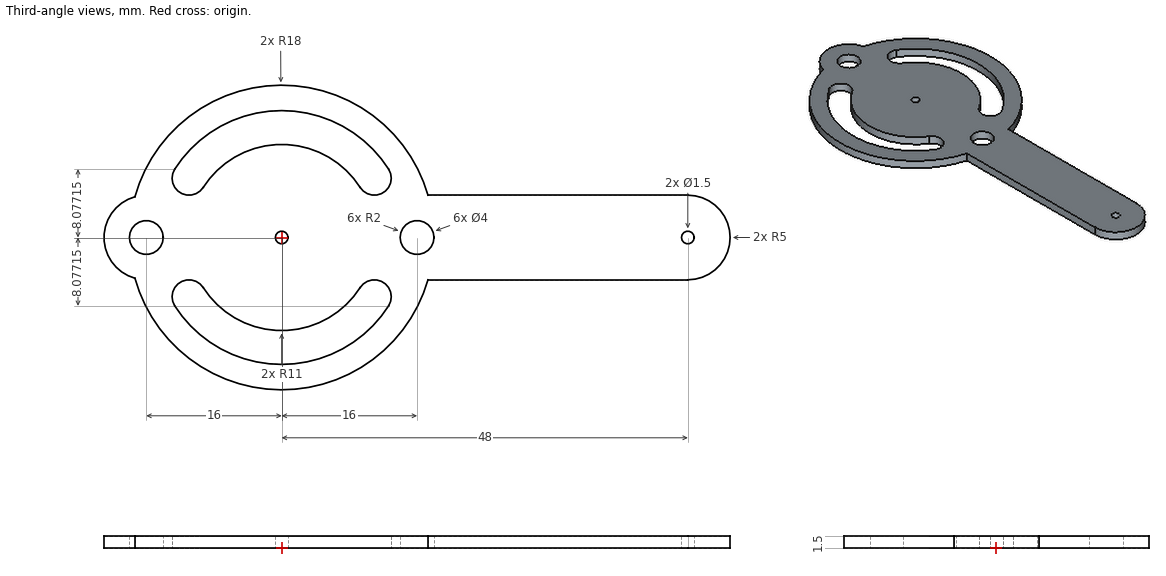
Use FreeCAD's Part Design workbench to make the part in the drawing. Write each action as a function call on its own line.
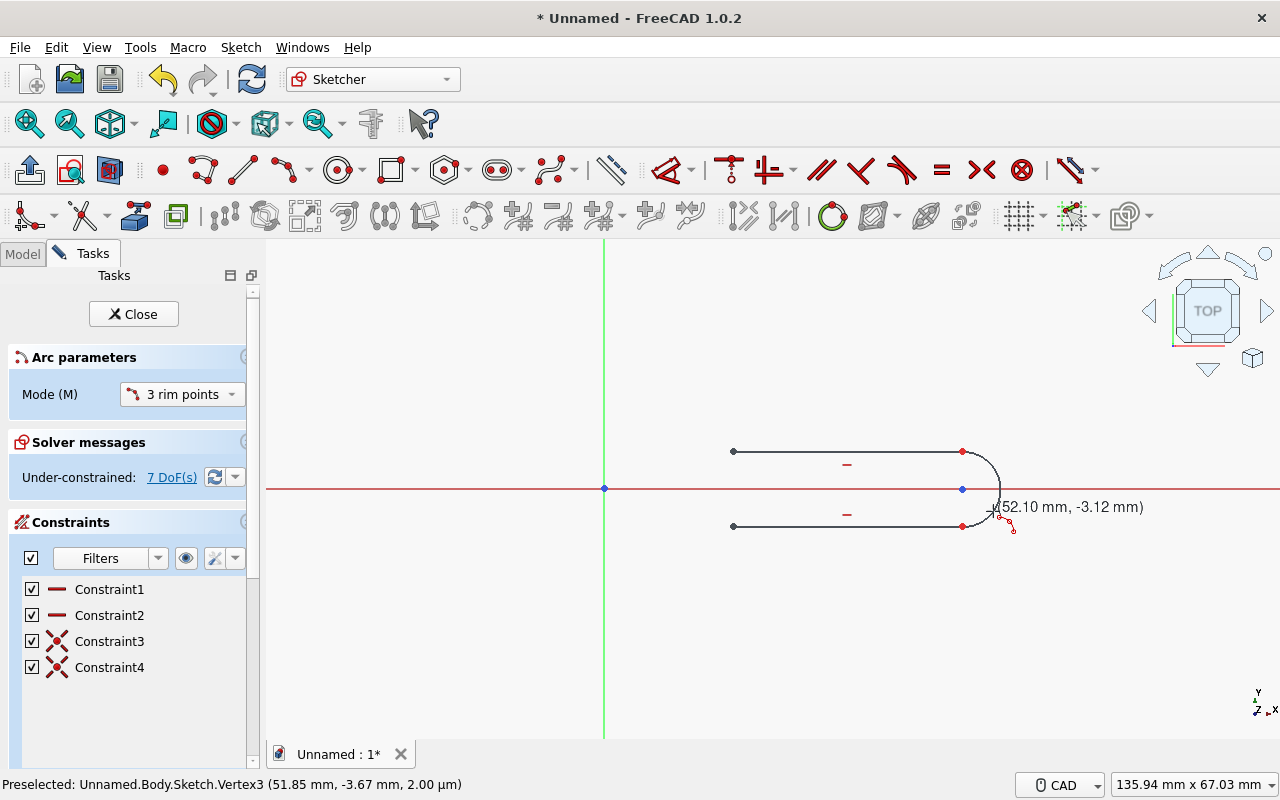
click(733, 452)
click(475, 453)
click(638, 359)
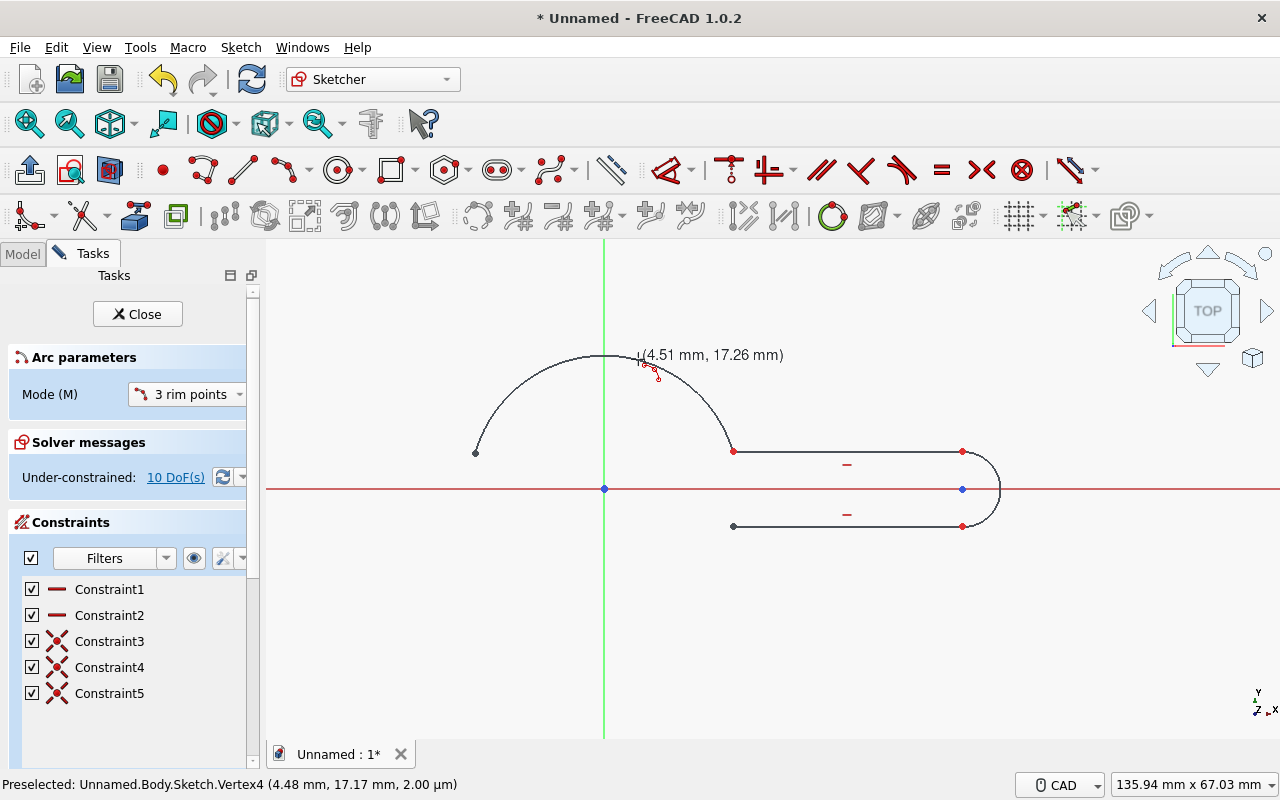
click(475, 454)
click(475, 525)
click(453, 470)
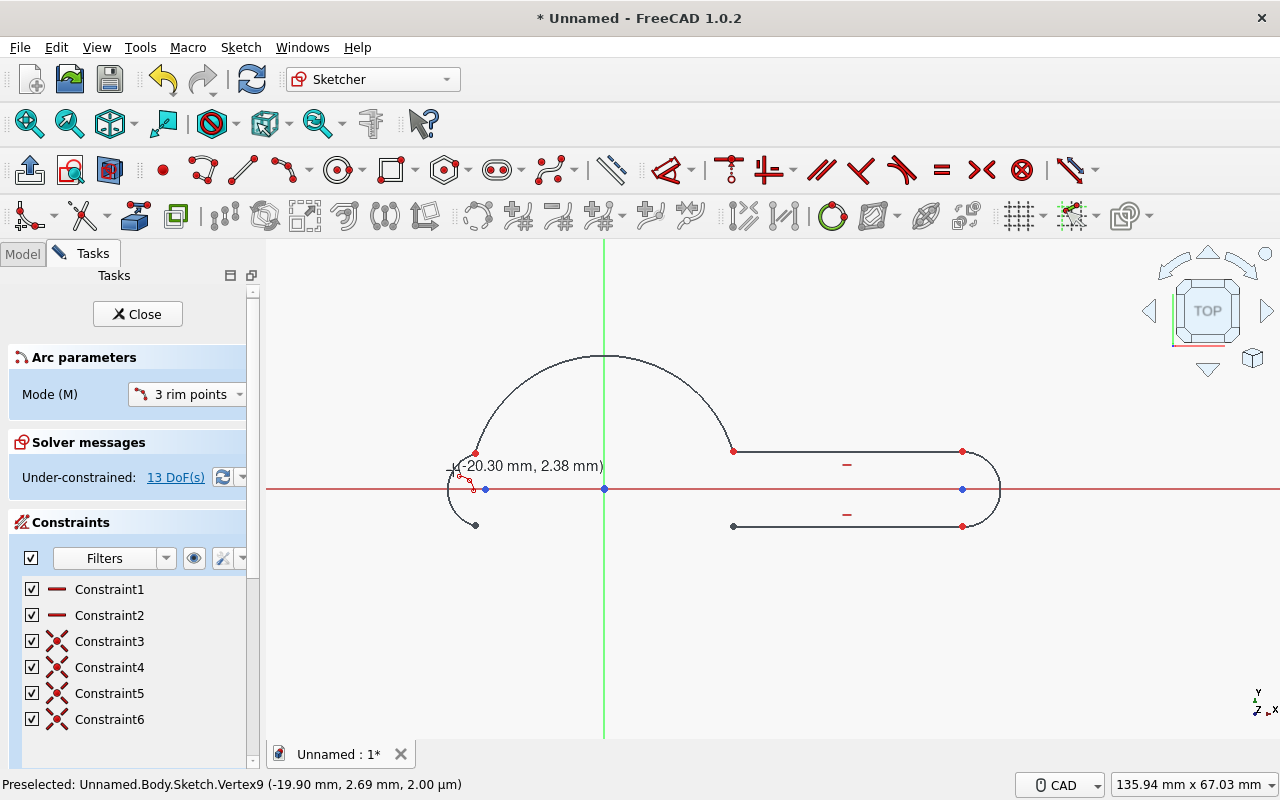
click(475, 526)
click(733, 527)
click(569, 618)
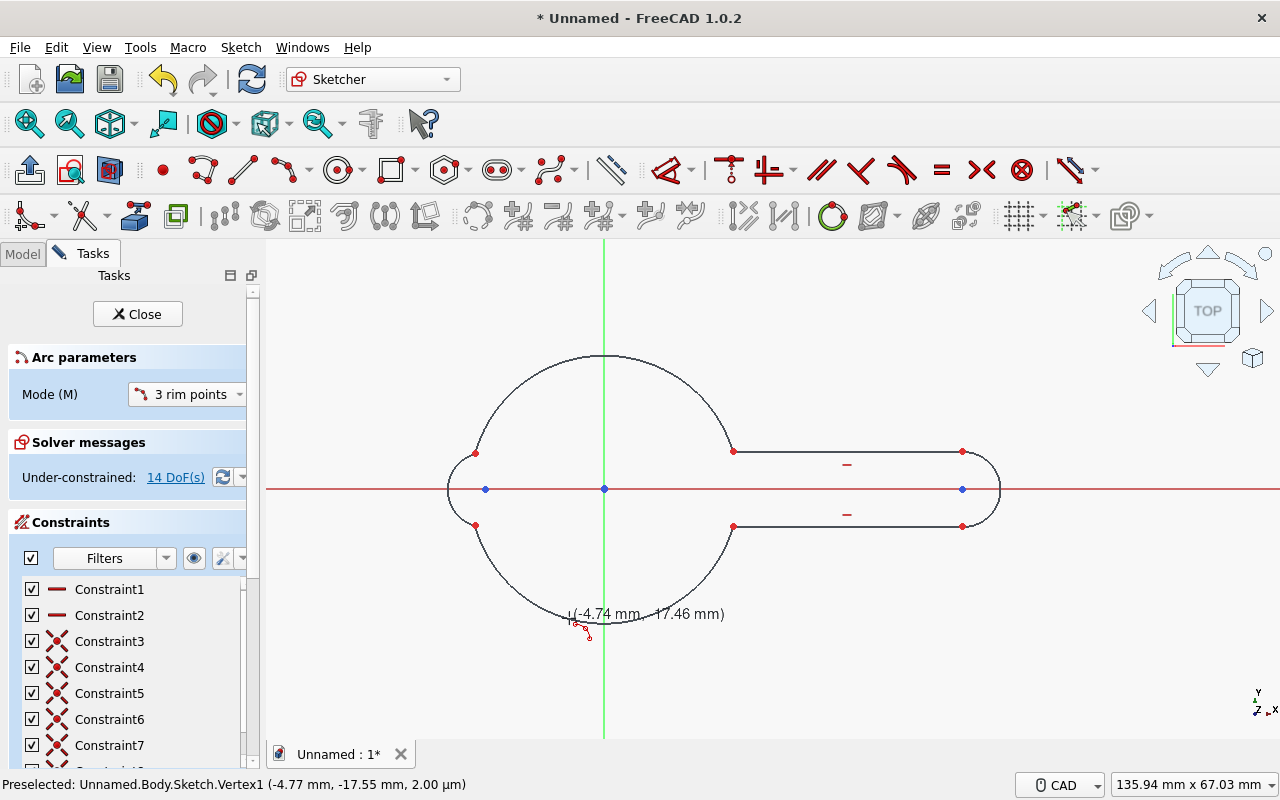
click(535, 533)
click(674, 533)
click(588, 569)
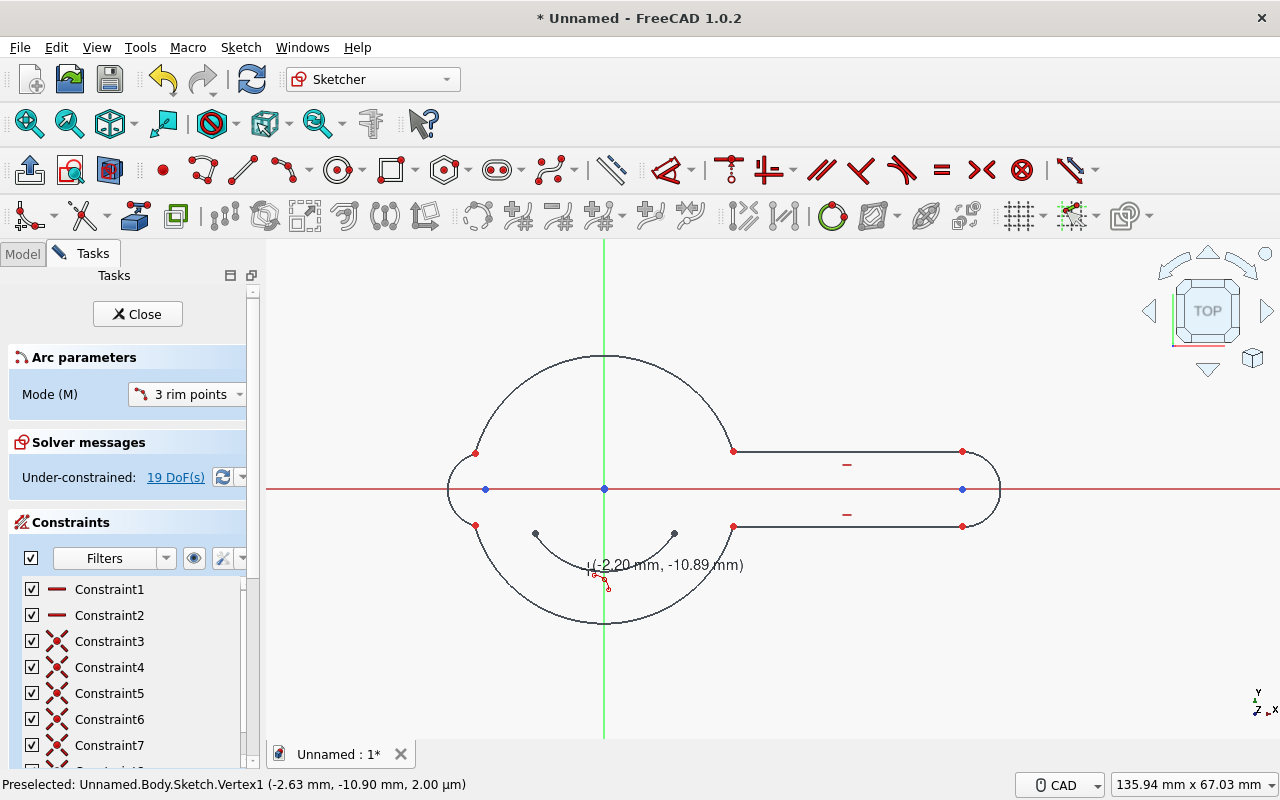
click(674, 534)
click(699, 549)
click(694, 528)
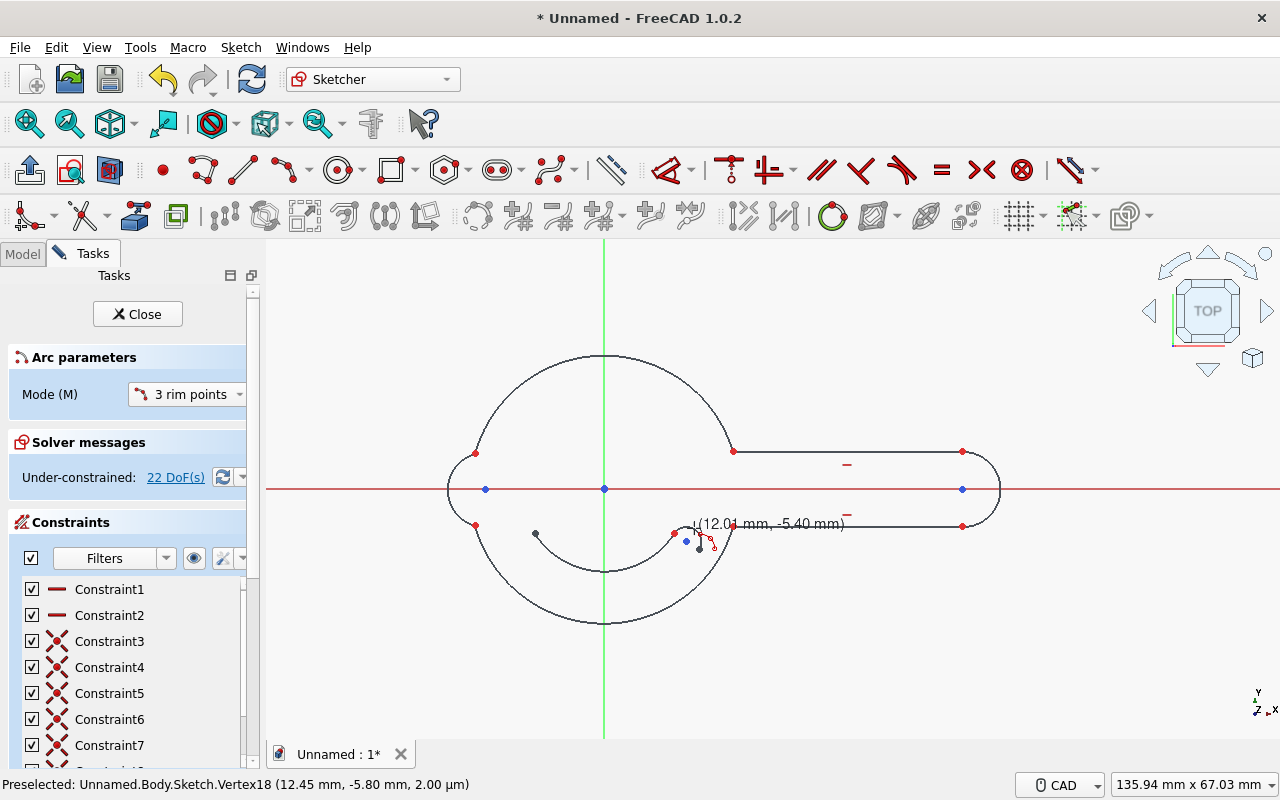
click(699, 550)
click(510, 549)
click(582, 598)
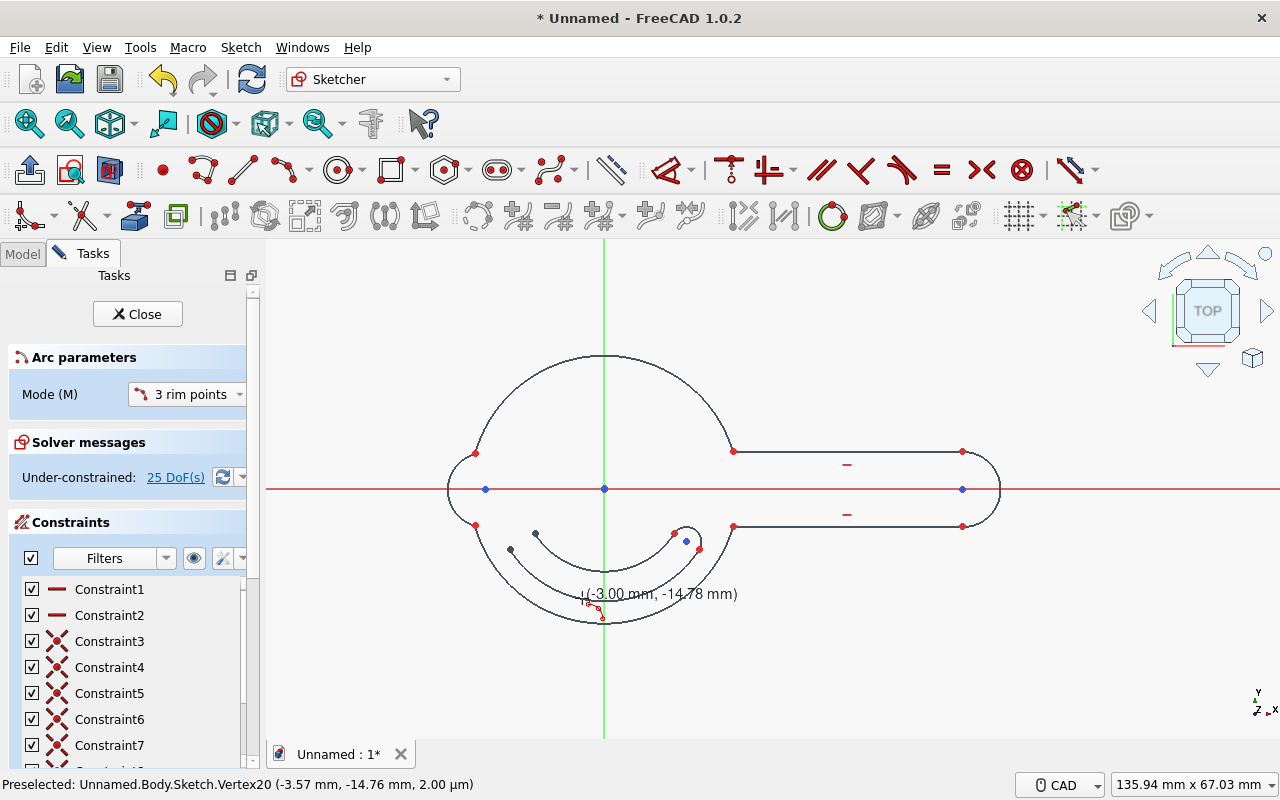
click(510, 550)
click(535, 534)
click(515, 528)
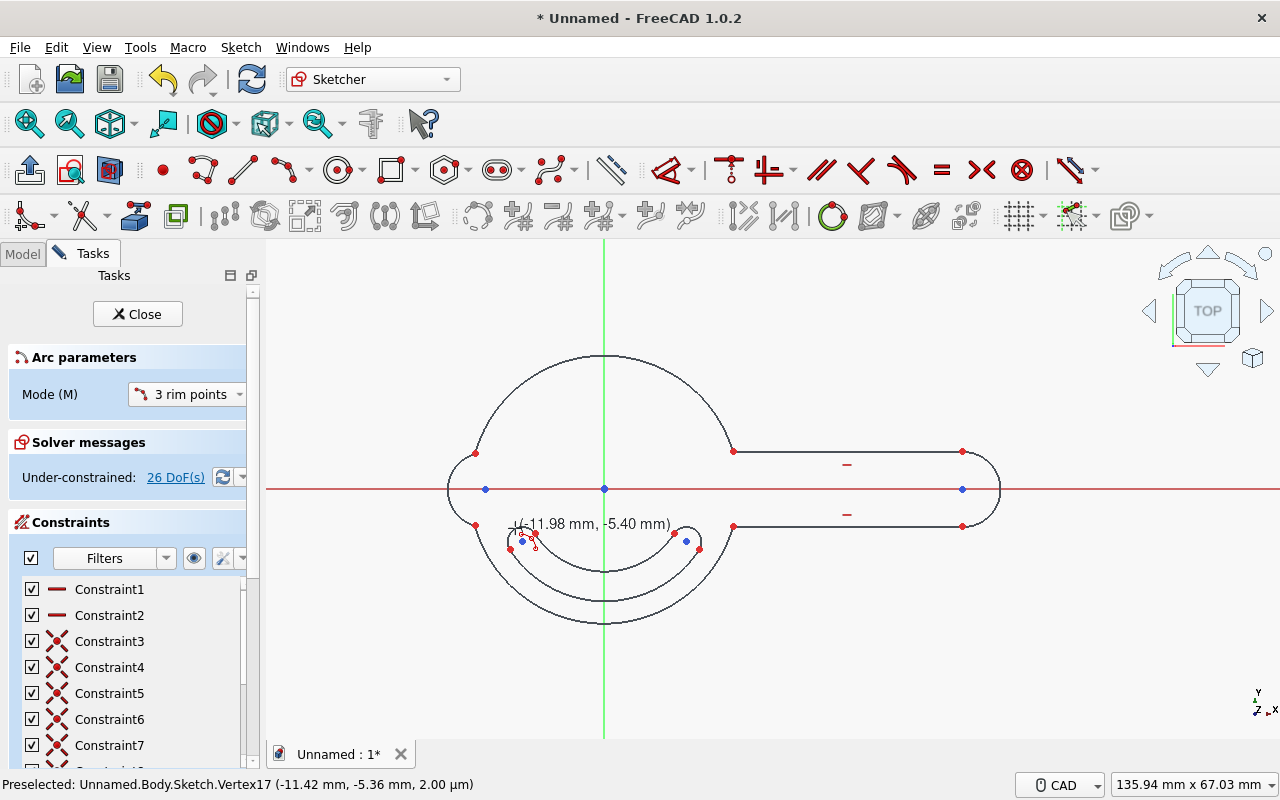
click(674, 445)
click(535, 445)
click(621, 408)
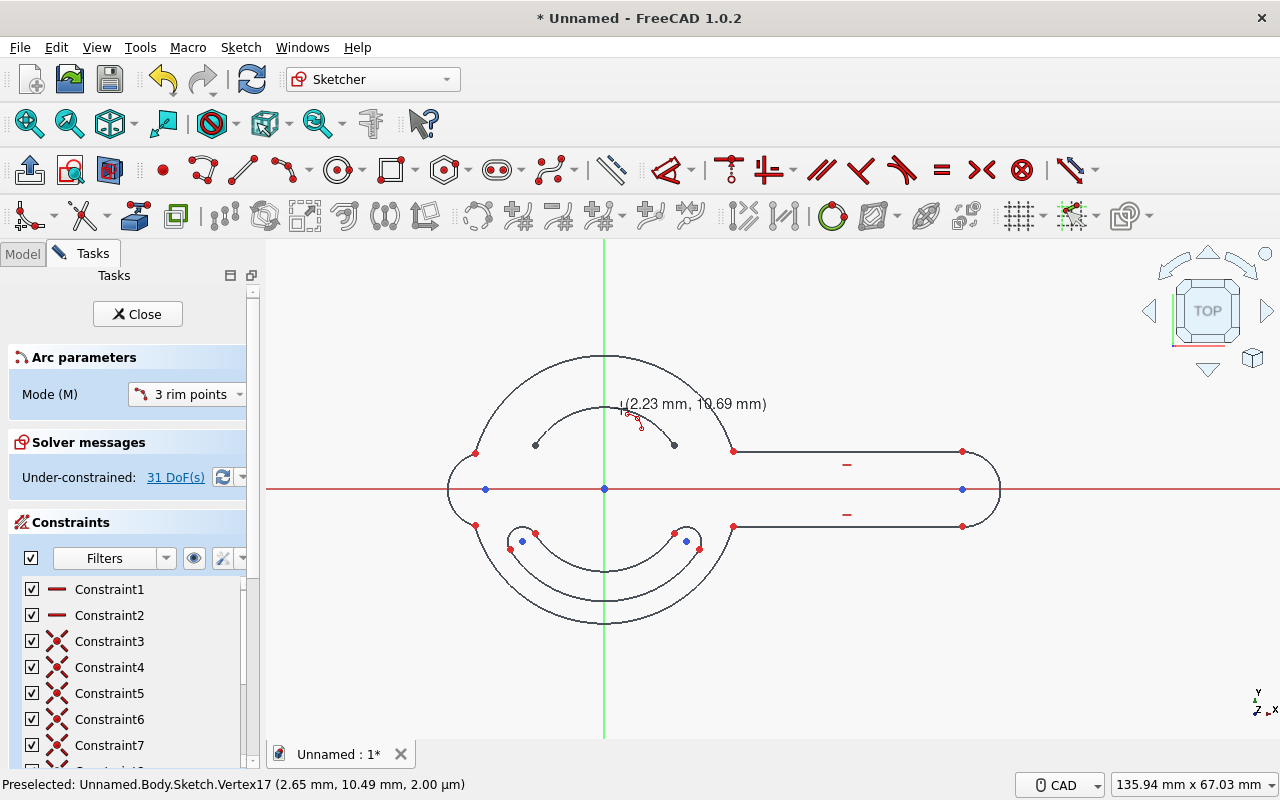
click(535, 446)
click(510, 429)
click(515, 449)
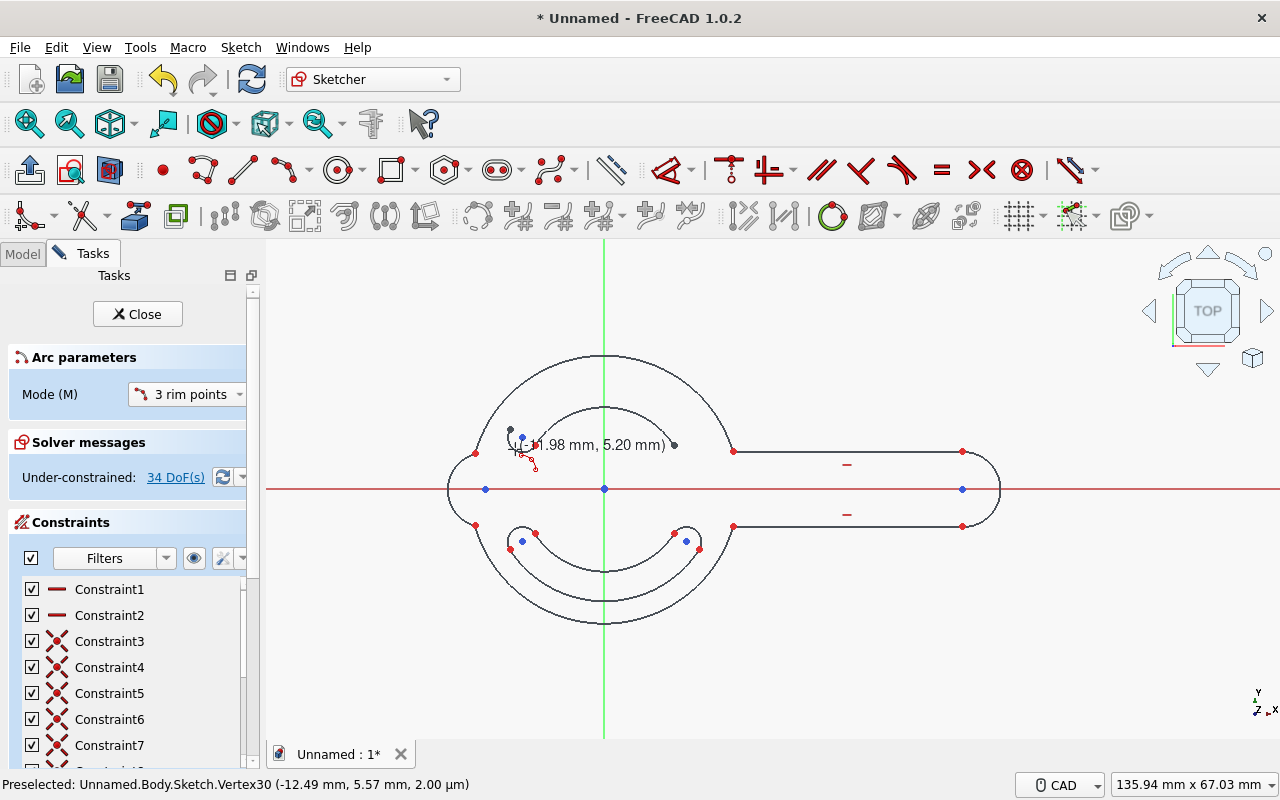
click(510, 430)
click(699, 429)
click(627, 379)